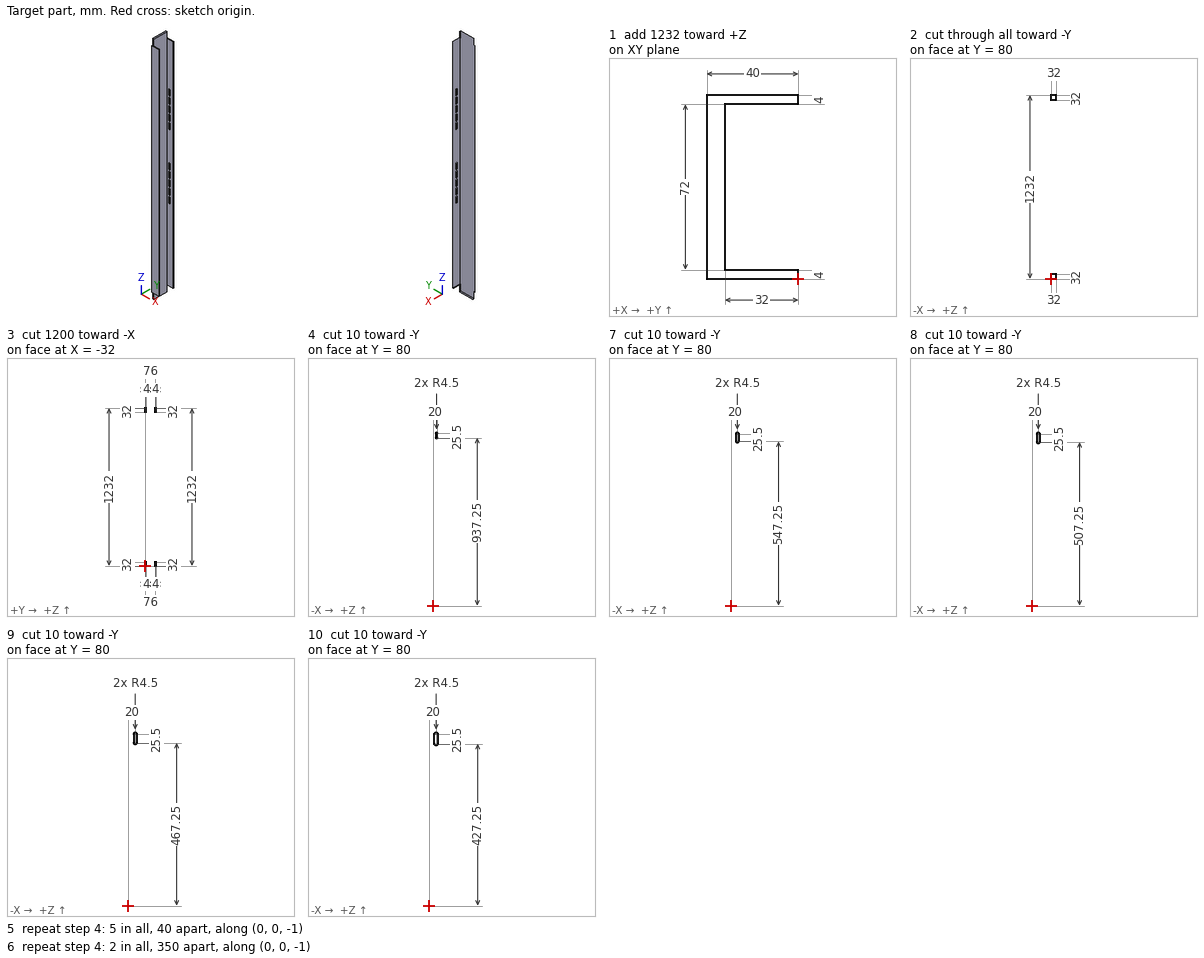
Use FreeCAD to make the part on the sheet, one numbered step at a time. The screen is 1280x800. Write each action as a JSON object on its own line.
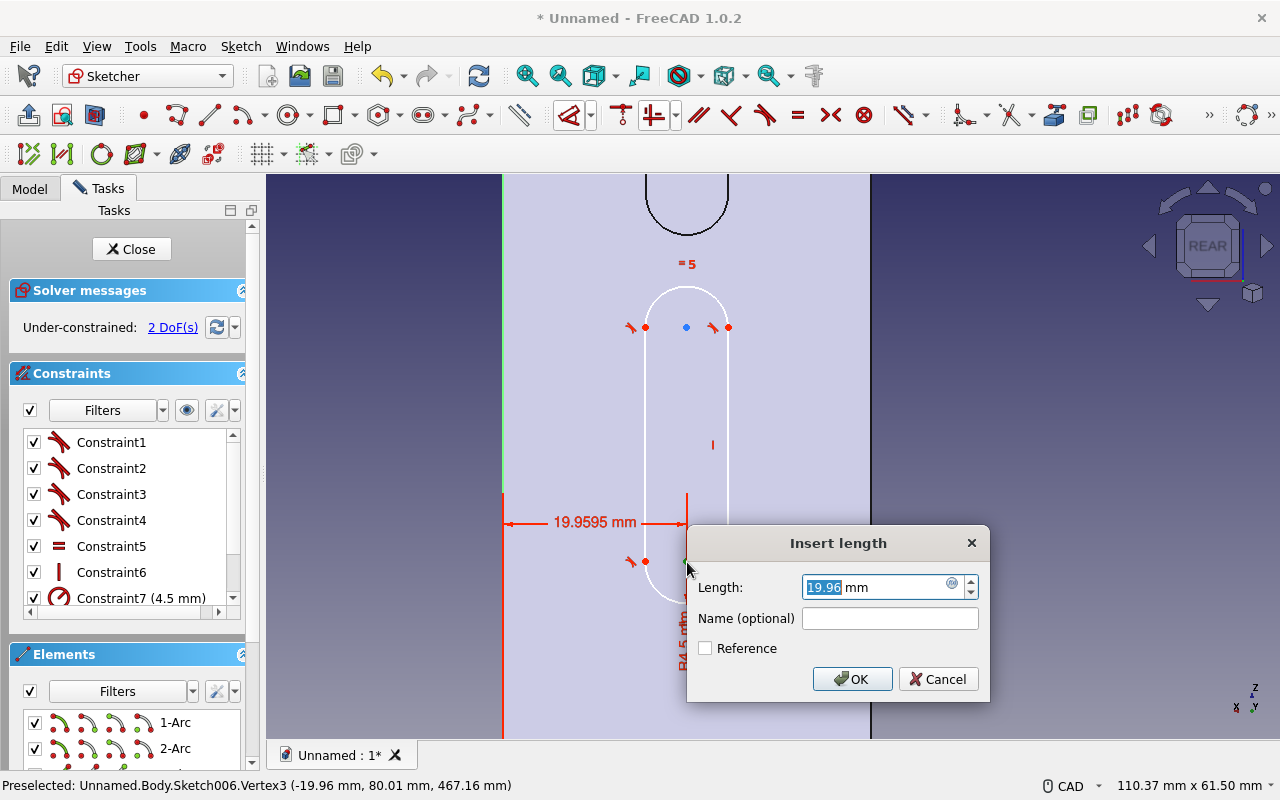
{"action": "type", "text": "20"}
{"action": "key", "text": "Return"}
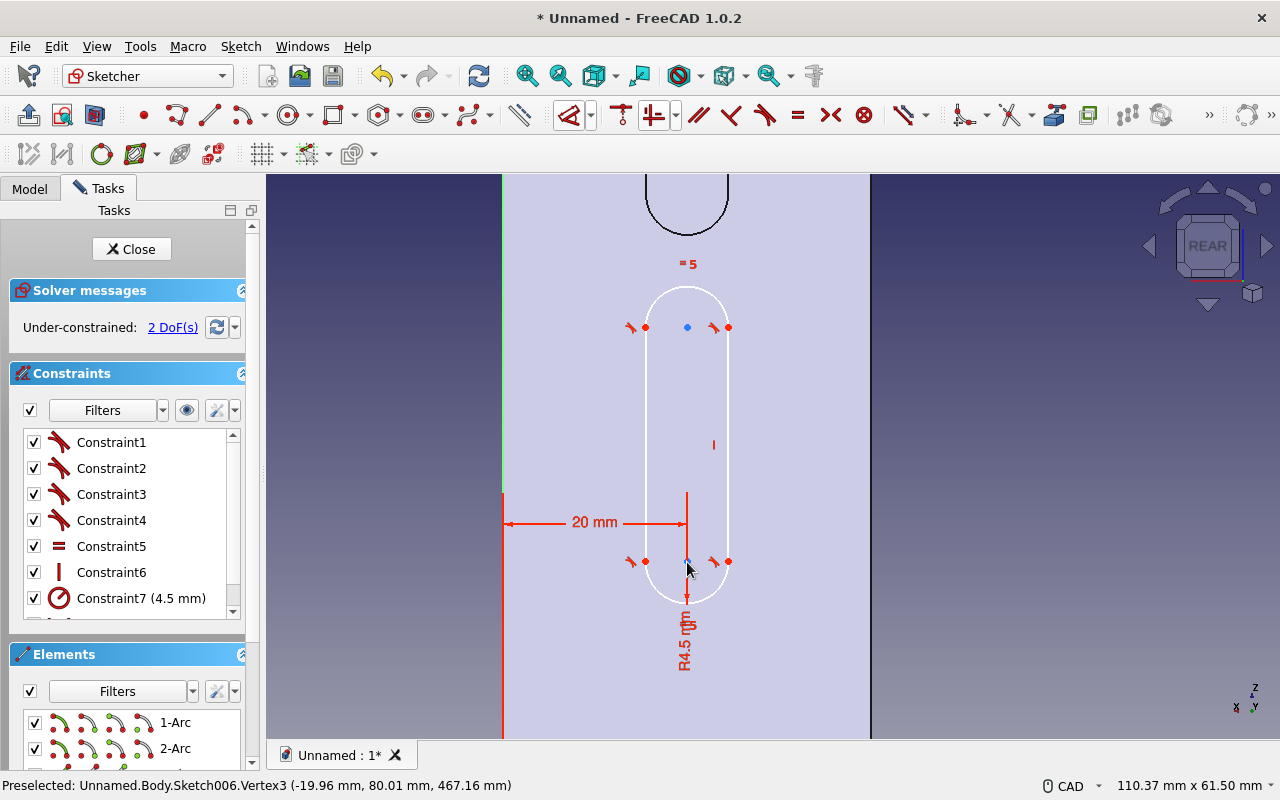
{"action": "left_click", "coordinate": [646, 492]}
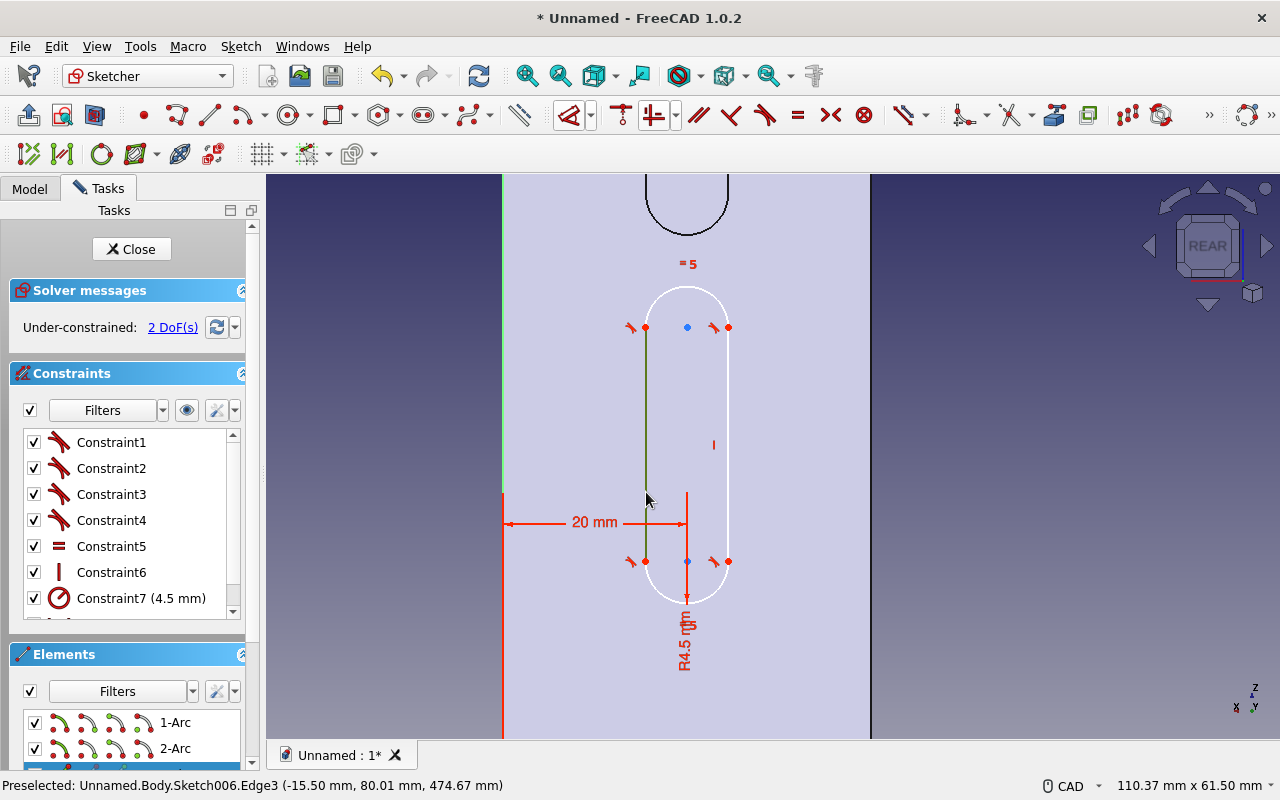
{"action": "left_click", "coordinate": [590, 116]}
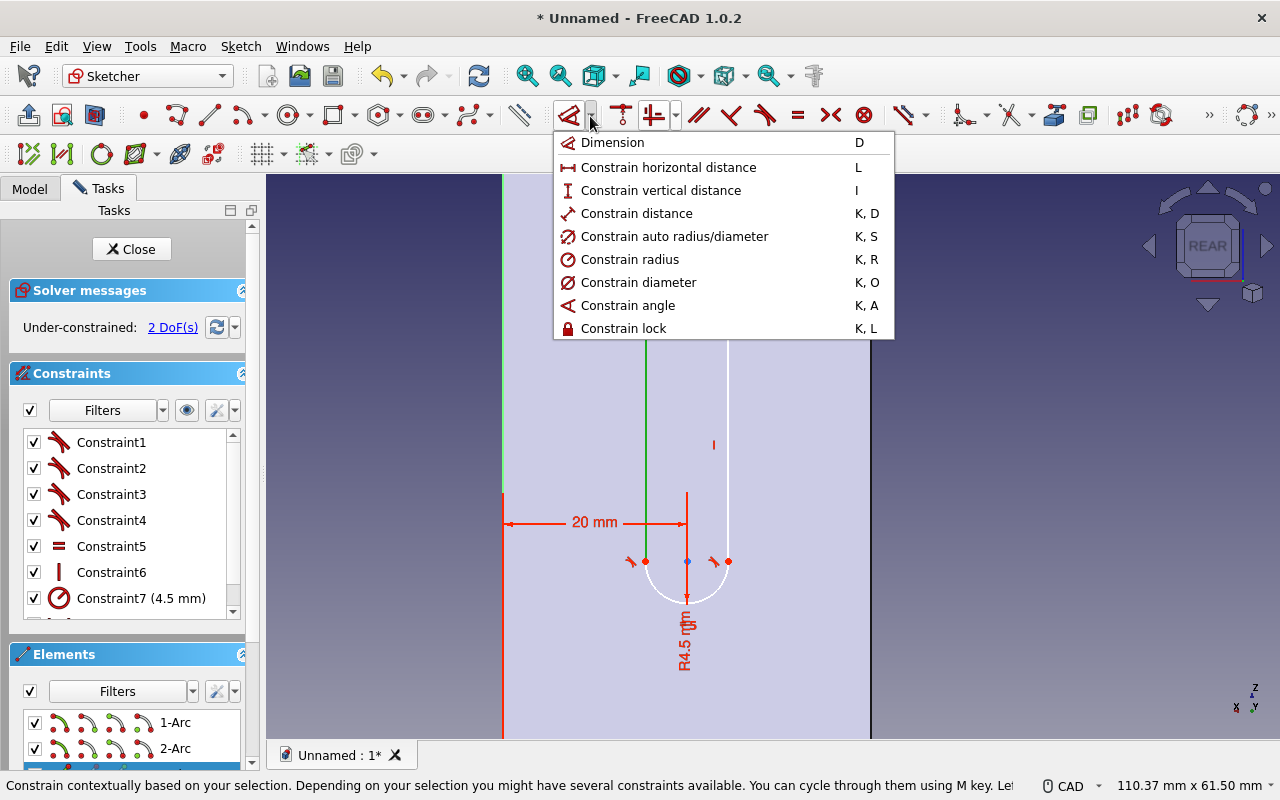
{"action": "left_click", "coordinate": [724, 190]}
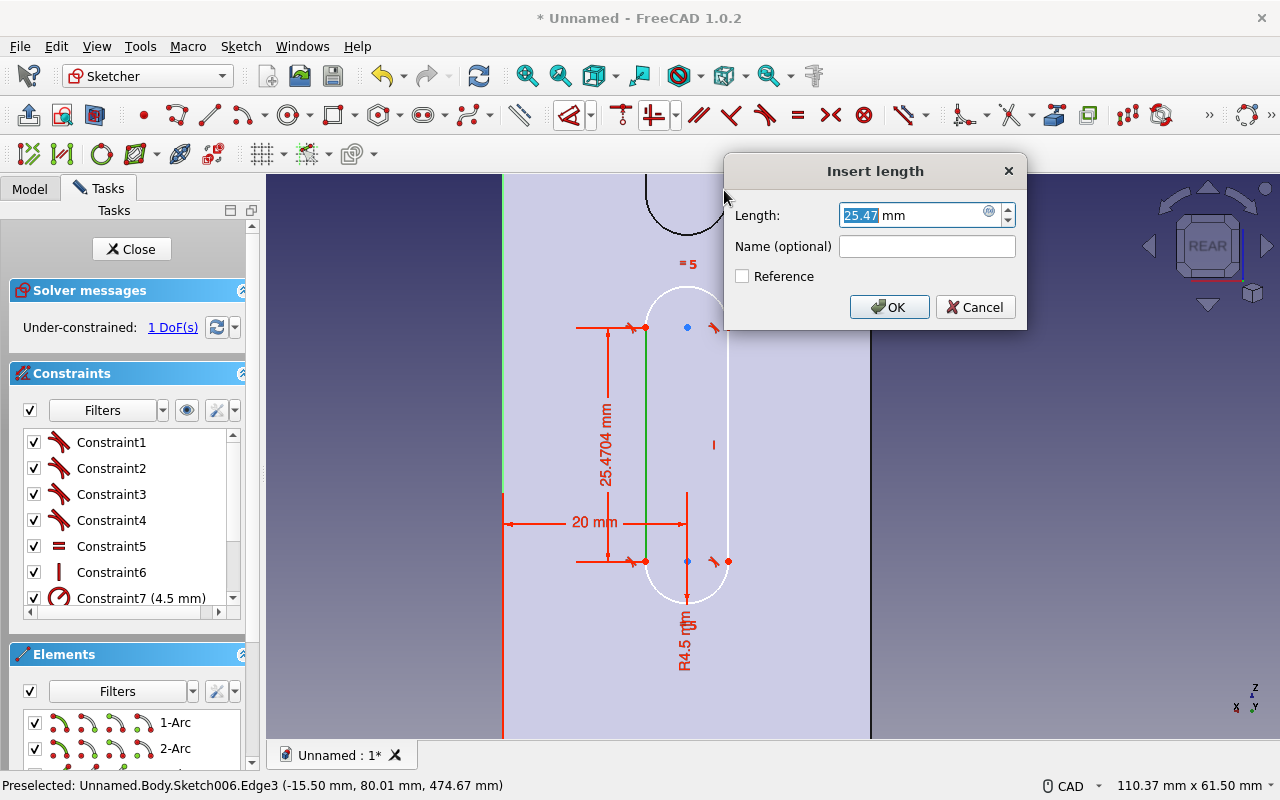
{"action": "type", "text": "25.5"}
{"action": "key", "text": "Return"}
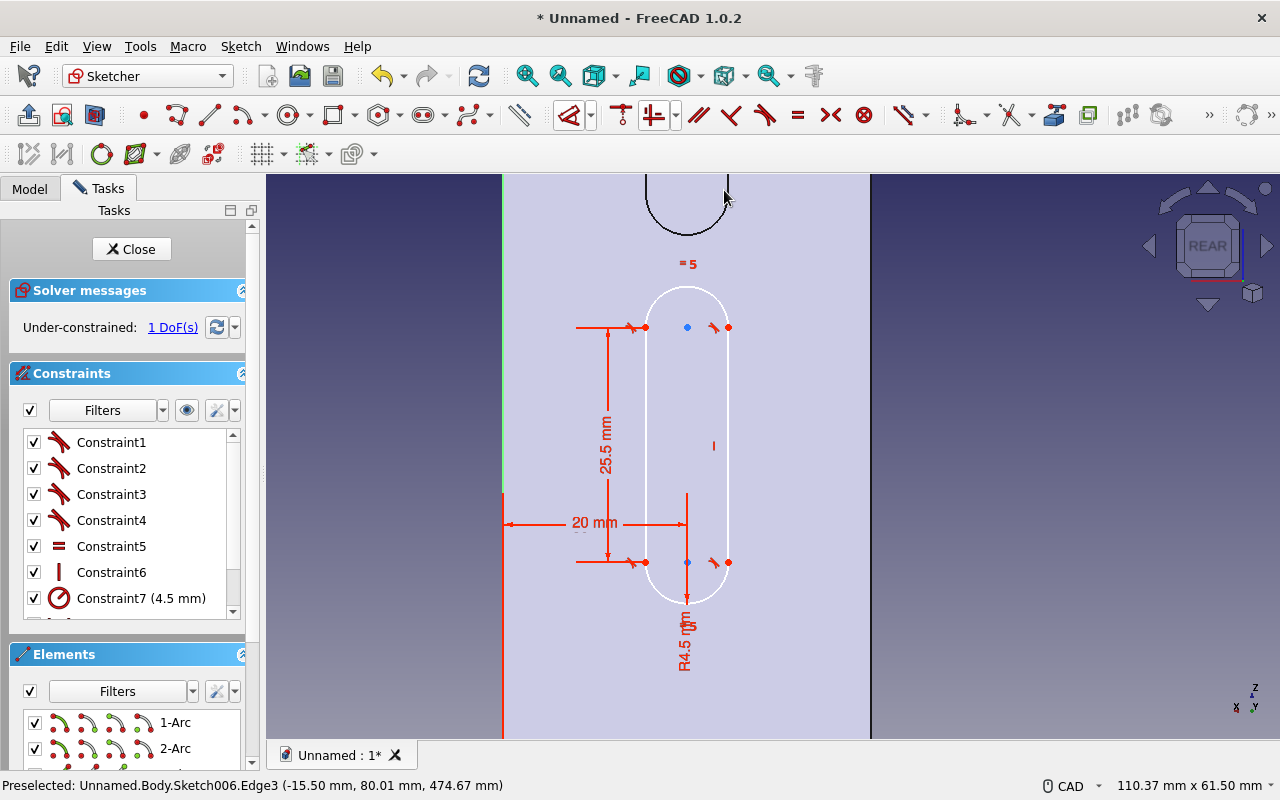
{"action": "left_click", "coordinate": [646, 562]}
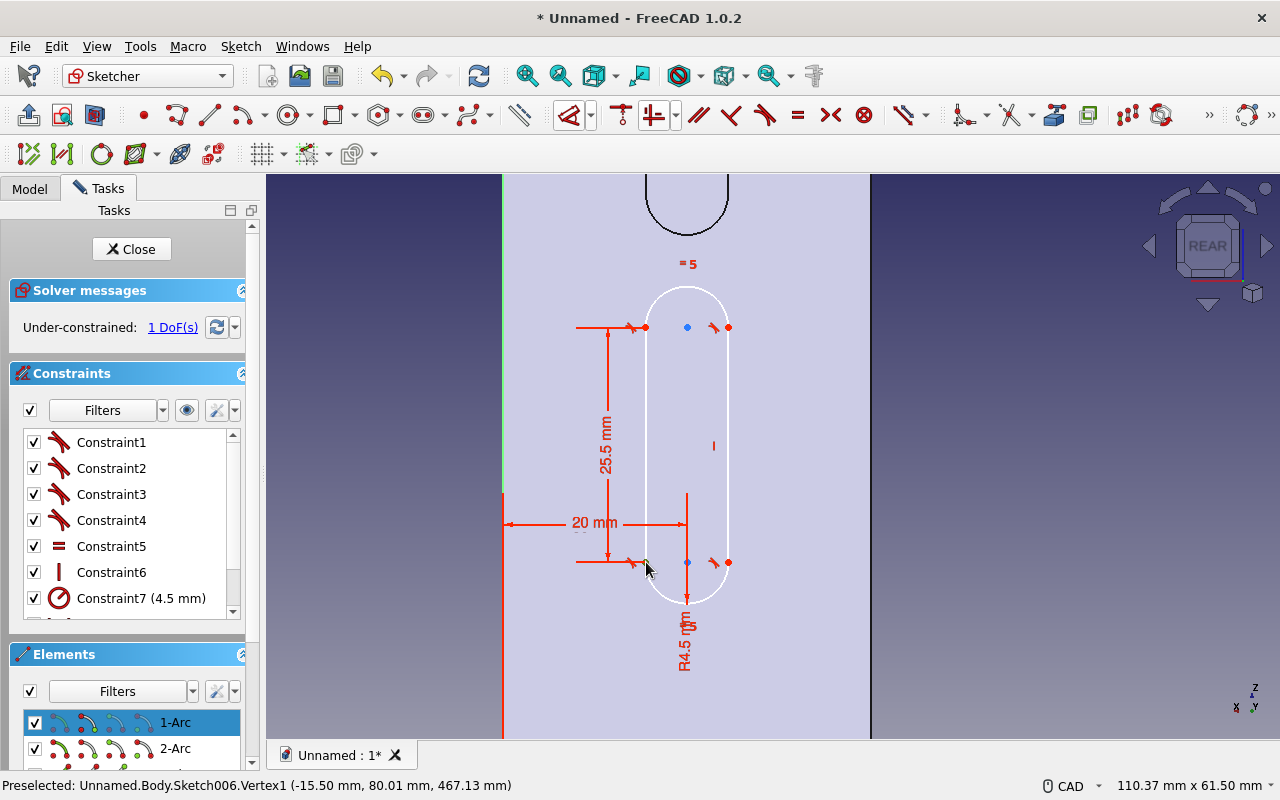
{"action": "key", "text": "i"}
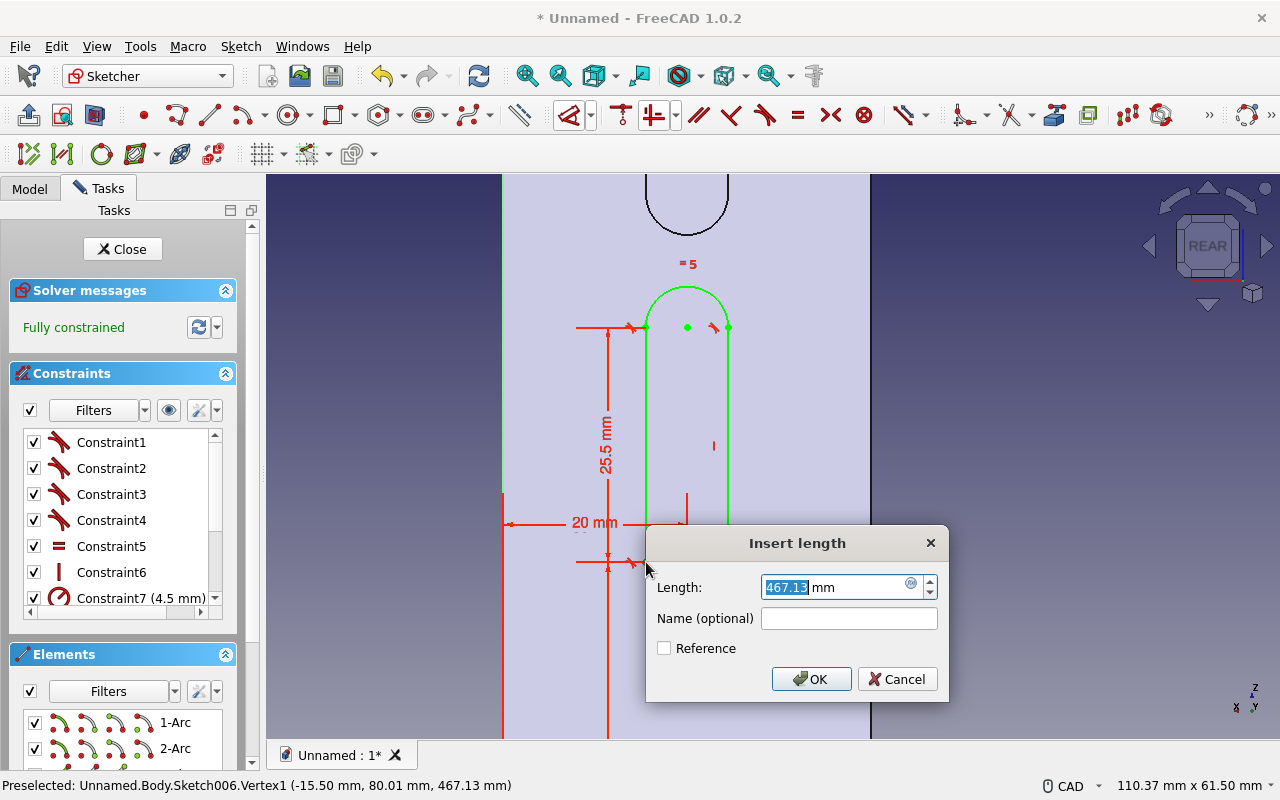
{"action": "type", "text": "467.25"}
{"action": "key", "text": "Return"}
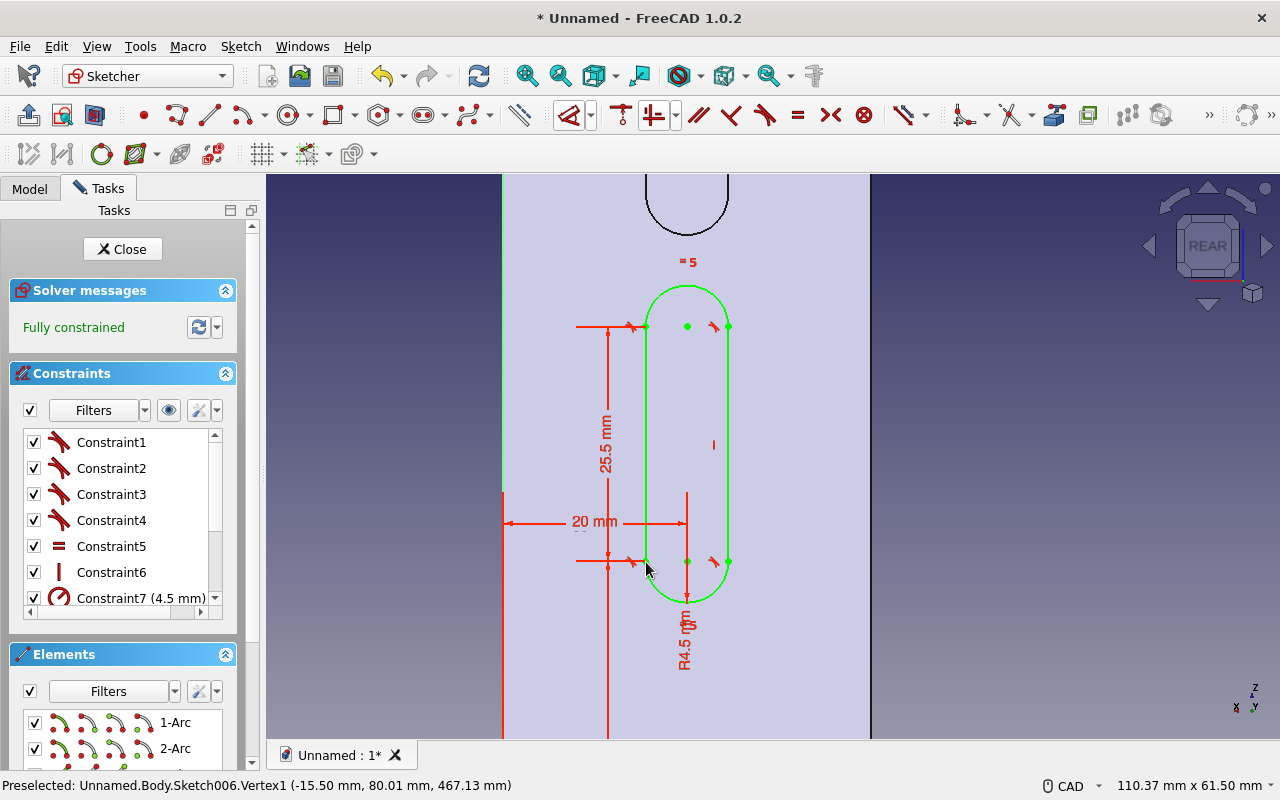
{"action": "left_click", "coordinate": [123, 249]}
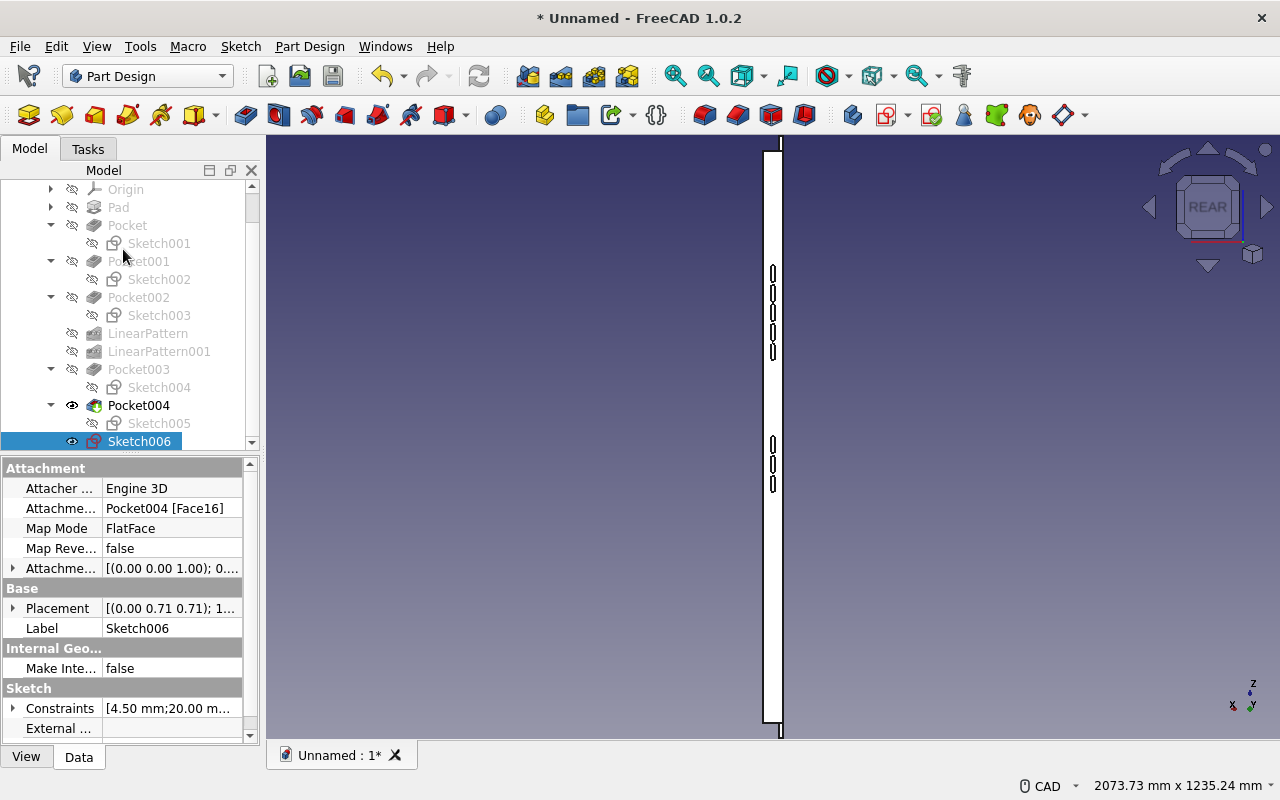
{"action": "left_click", "coordinate": [246, 116]}